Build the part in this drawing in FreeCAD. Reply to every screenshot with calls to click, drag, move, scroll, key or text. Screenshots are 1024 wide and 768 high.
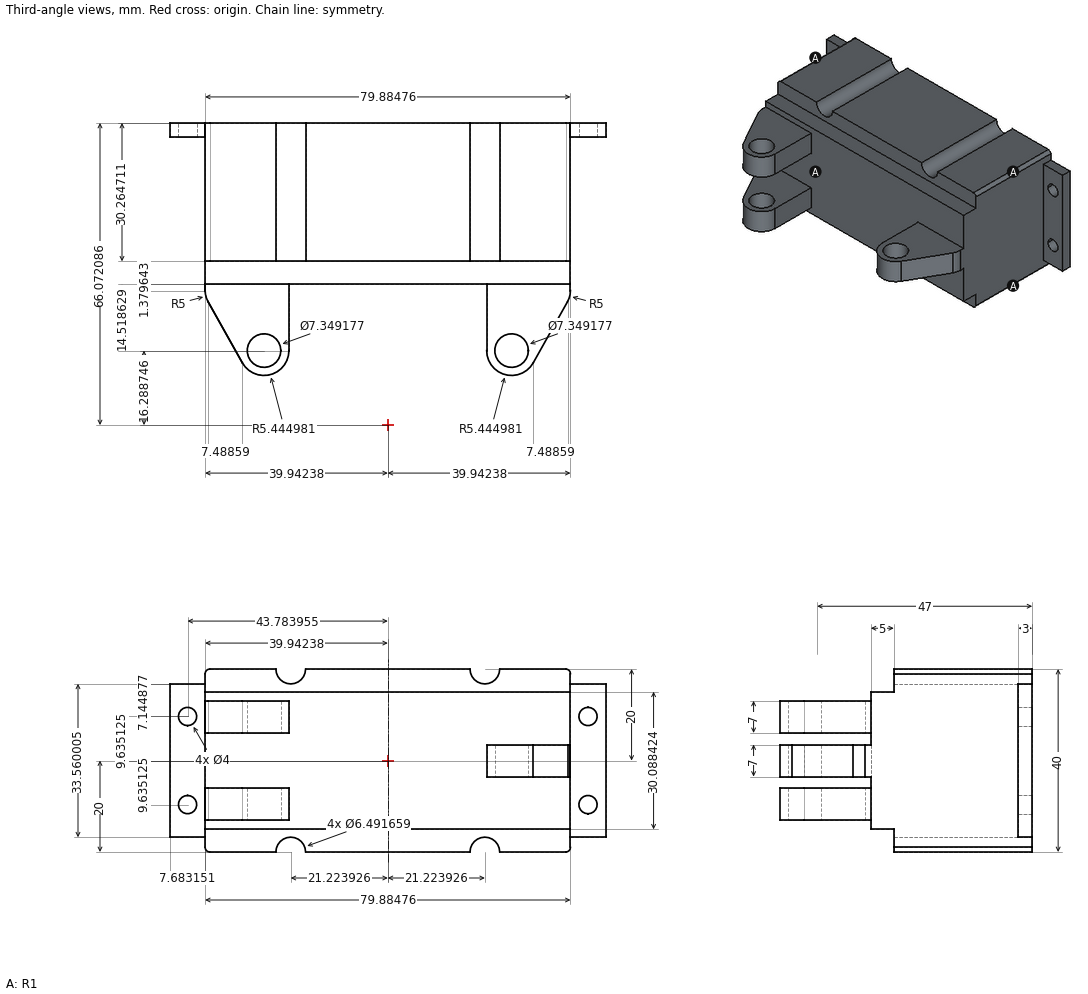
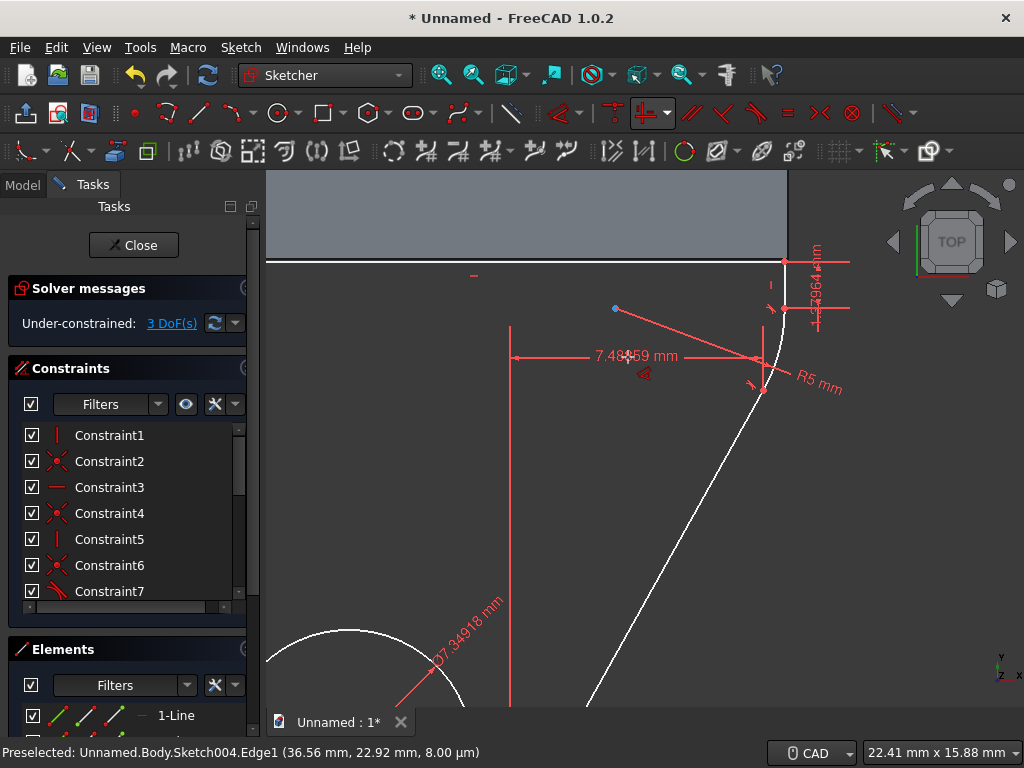
scroll(777, 291, down, 6)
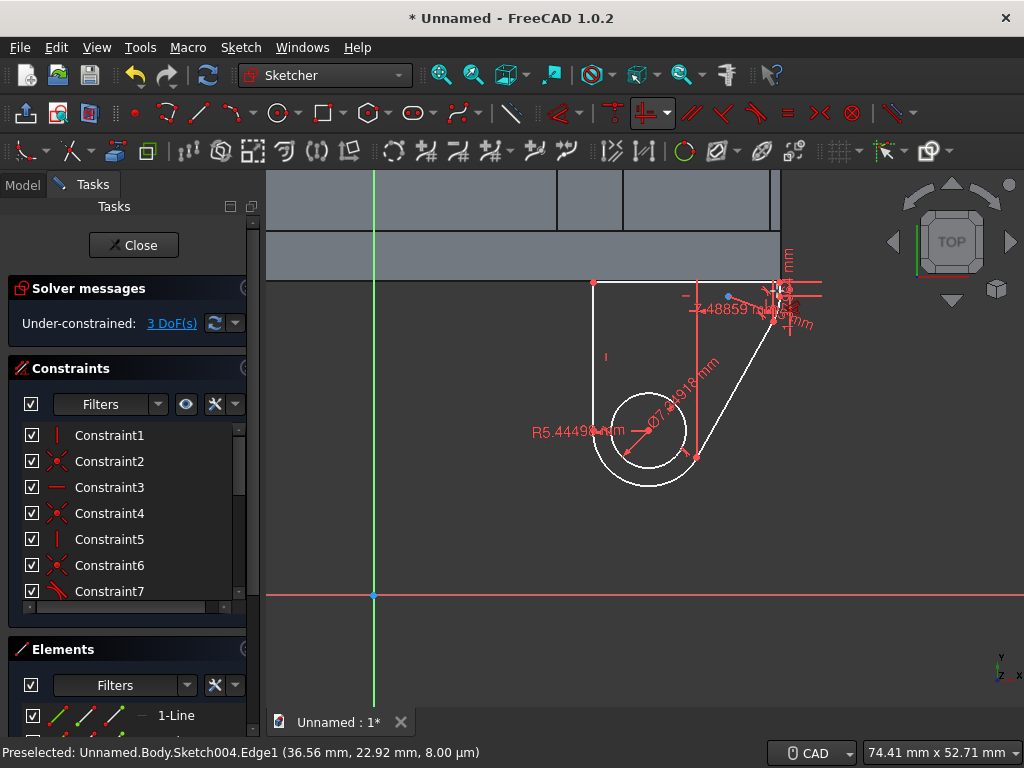
click(593, 327)
click(627, 356)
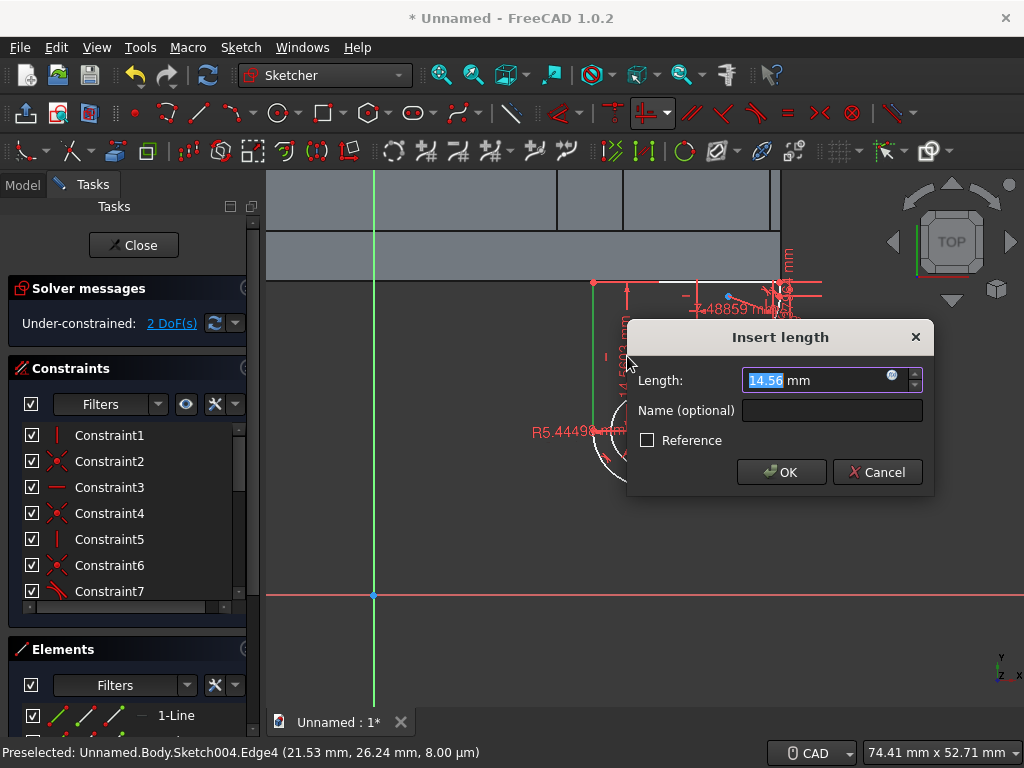
text(14.518629)
key(Return)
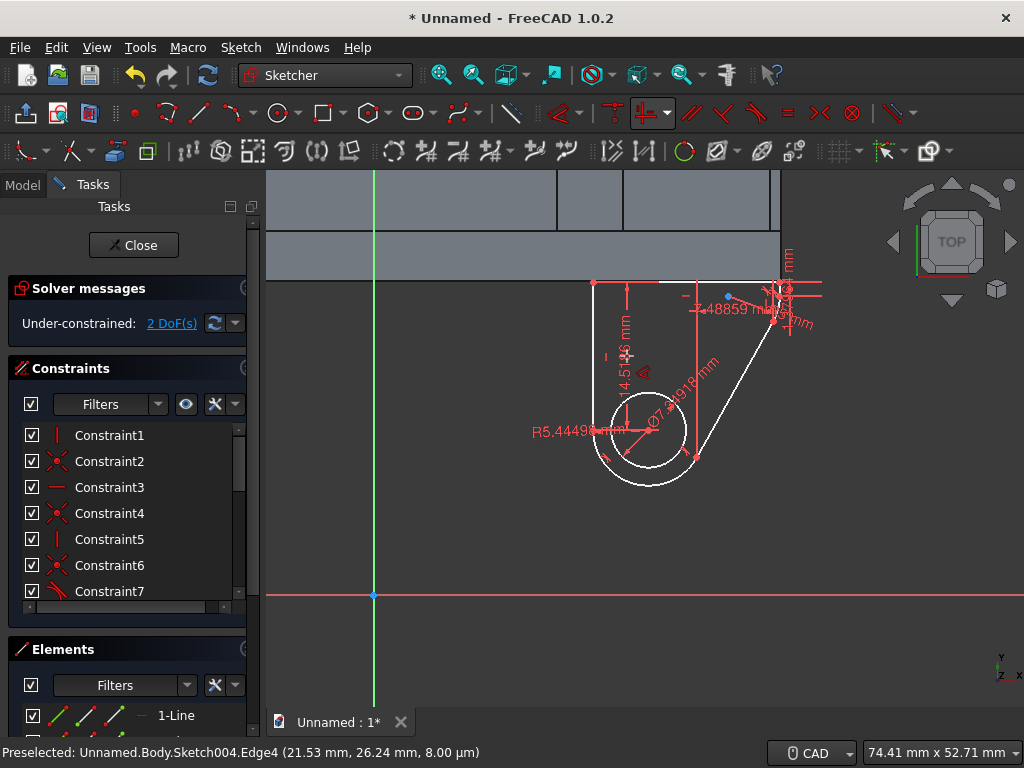
click(780, 296)
click(577, 629)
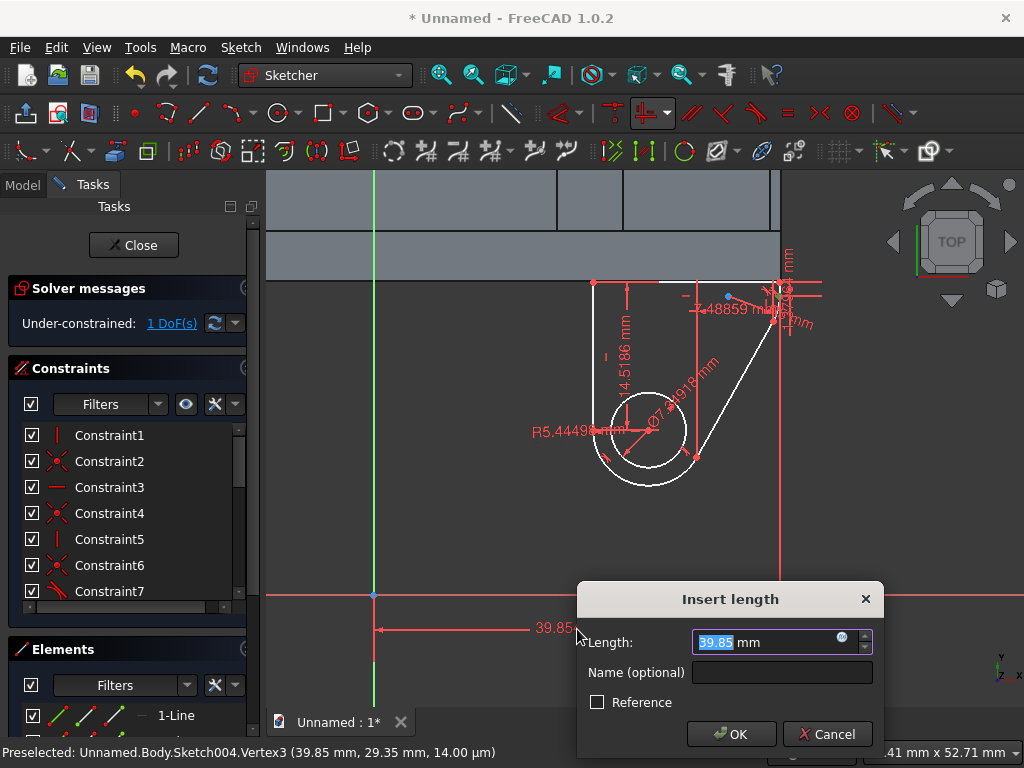
text(39.94238)
key(Return)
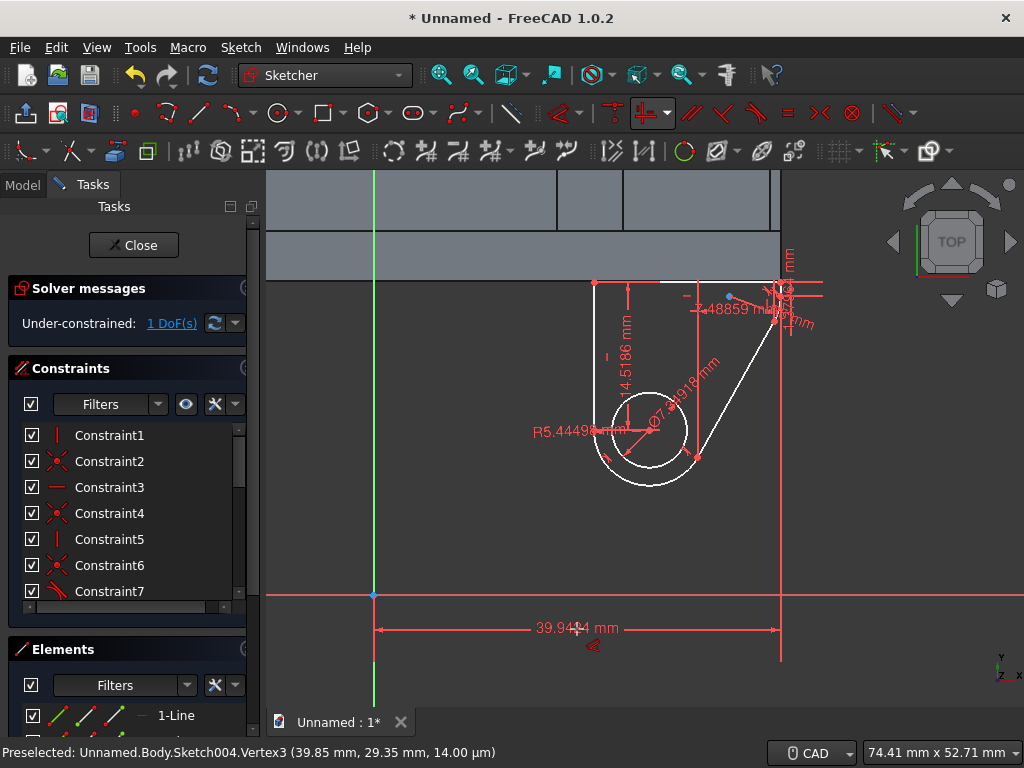
click(650, 430)
click(340, 513)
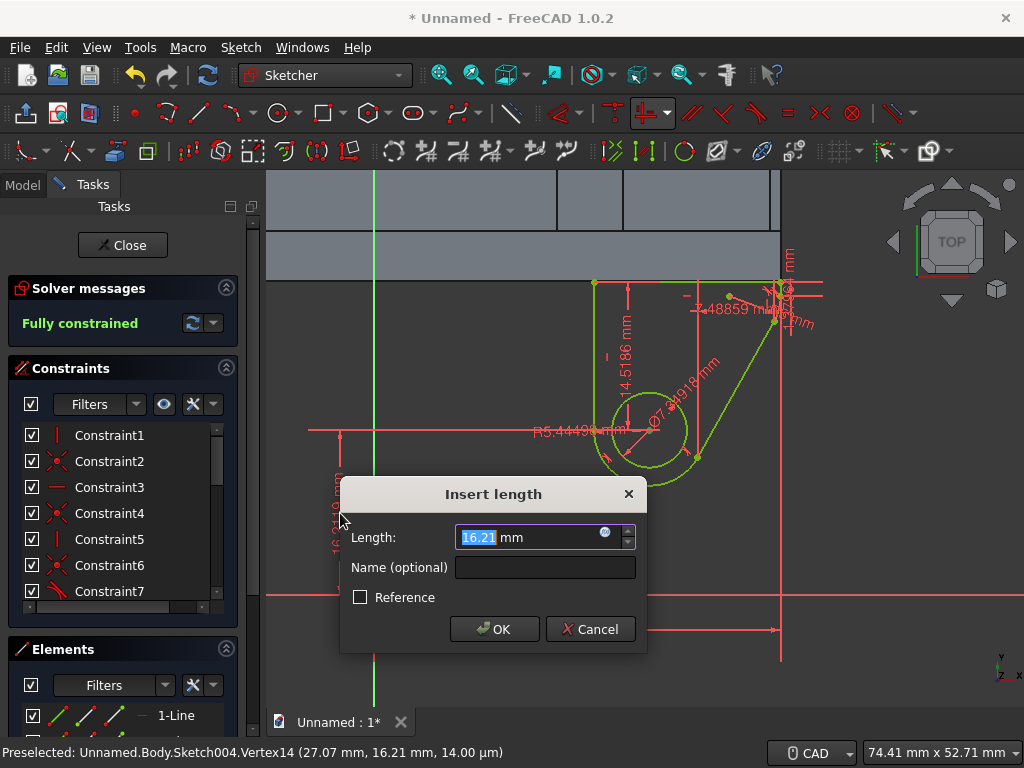
text(16.288746)
key(Return)
key(Escape)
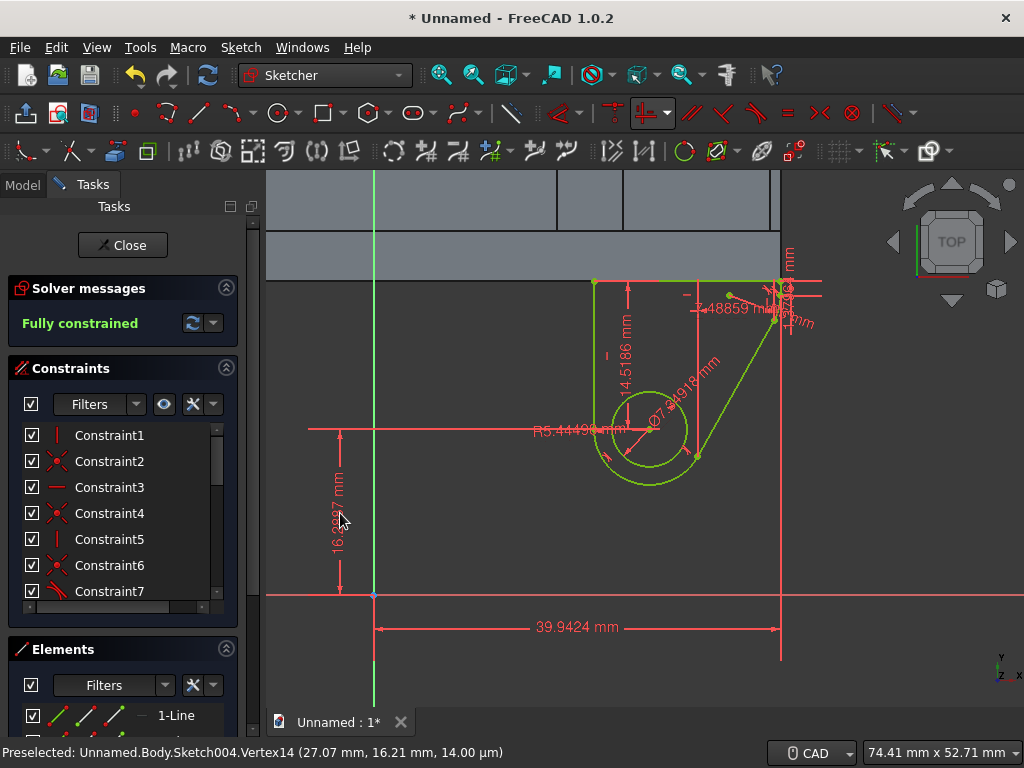
click(123, 245)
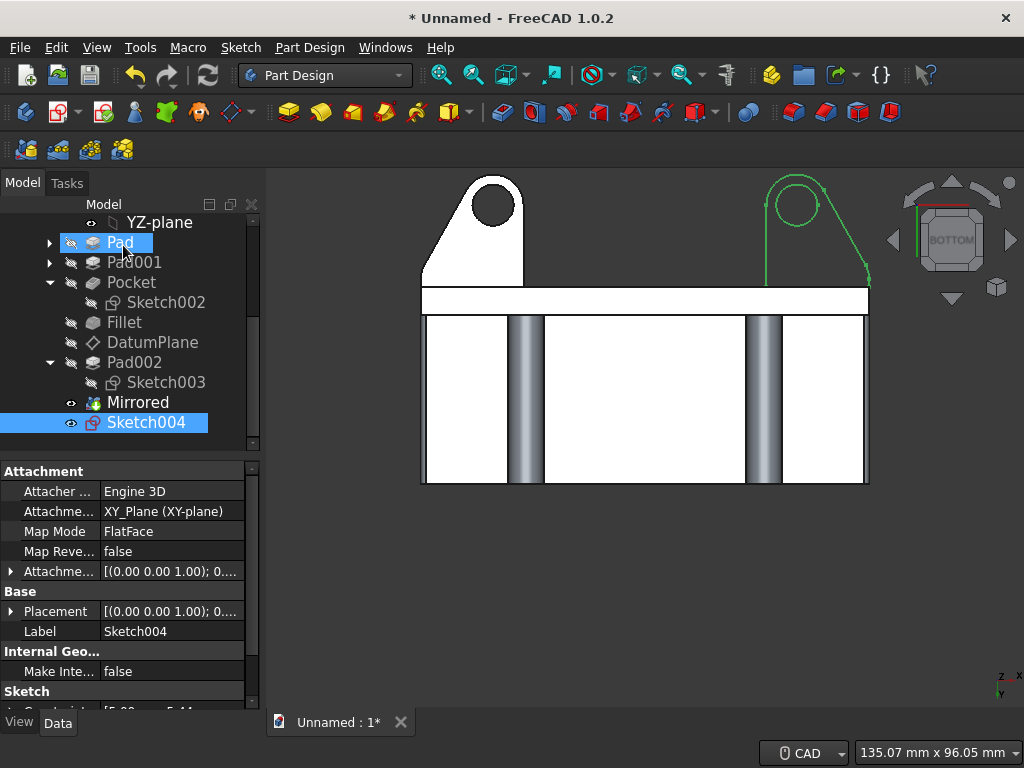
click(290, 112)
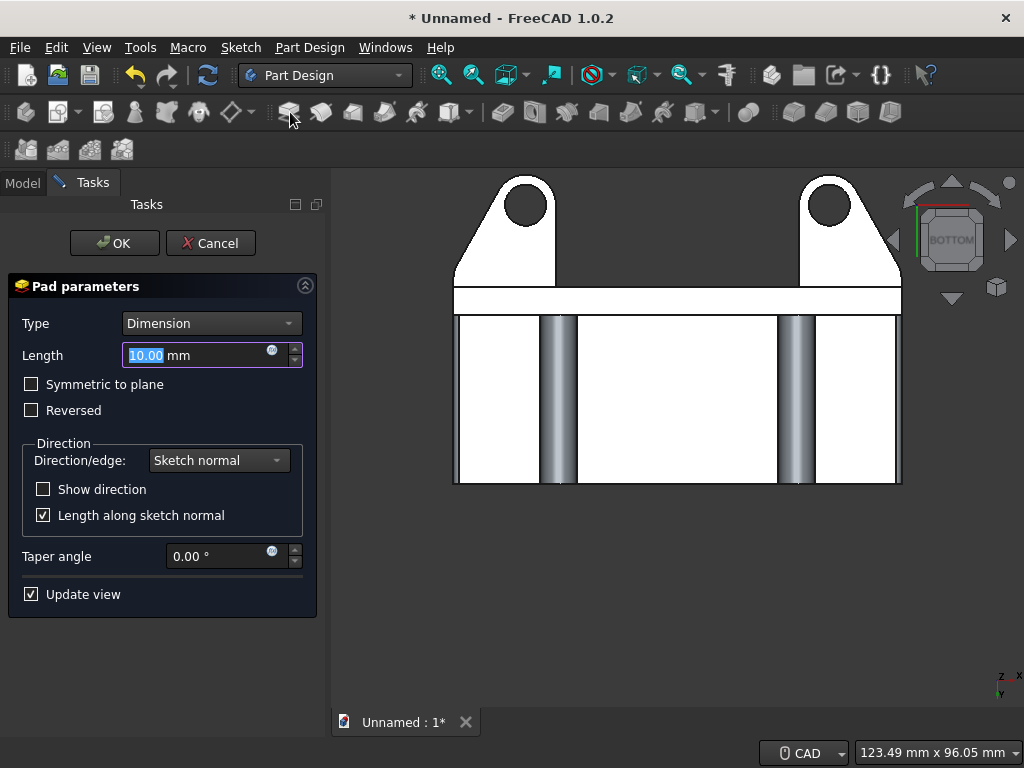
text(7)
key(Tab)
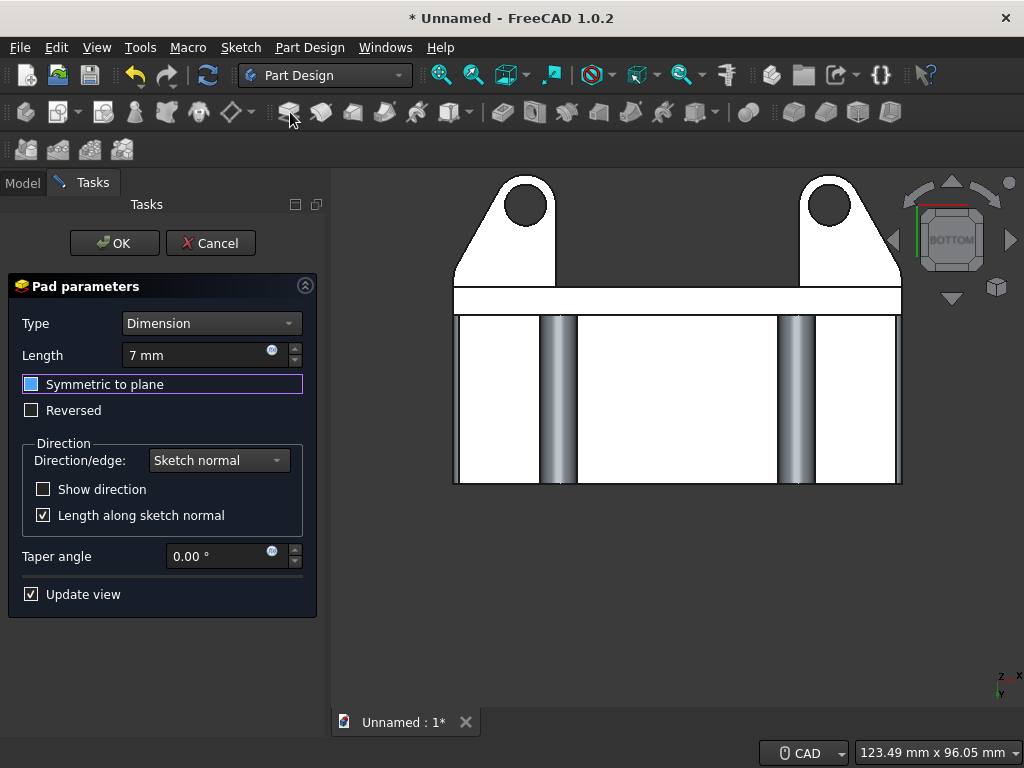
click(30, 384)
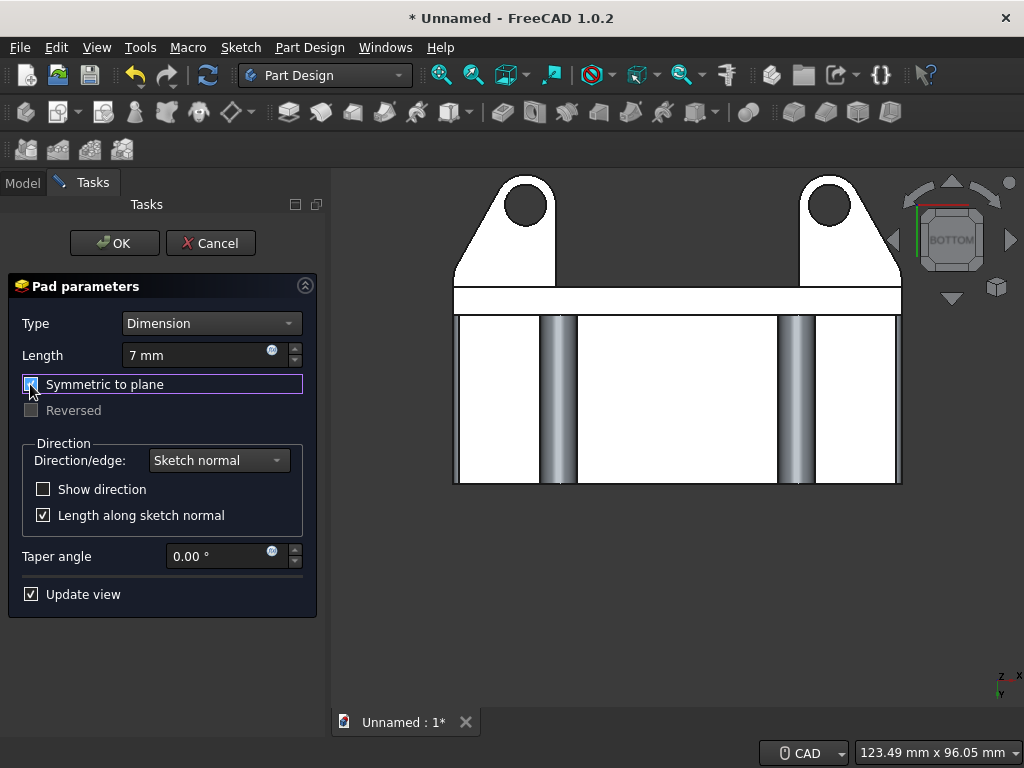
click(115, 243)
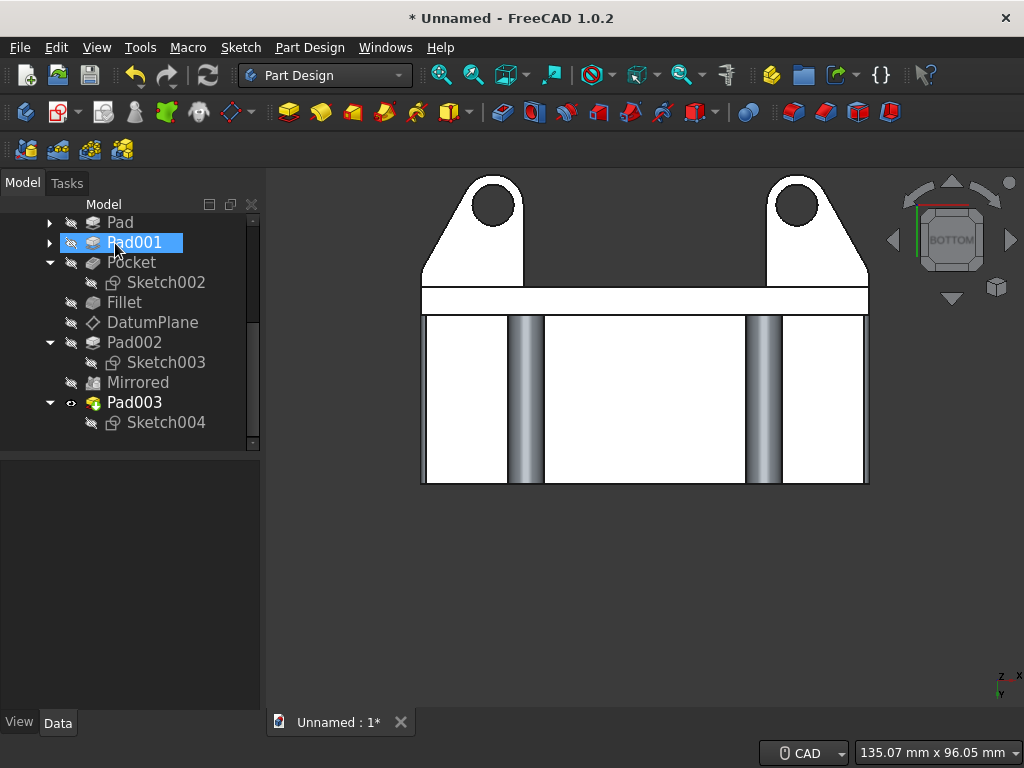
key(4)